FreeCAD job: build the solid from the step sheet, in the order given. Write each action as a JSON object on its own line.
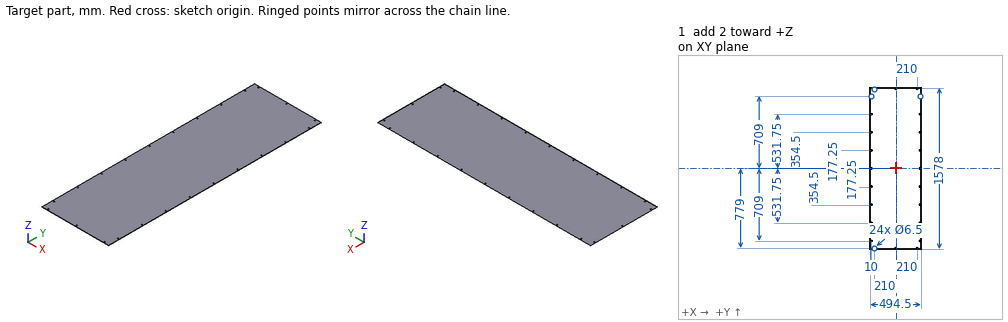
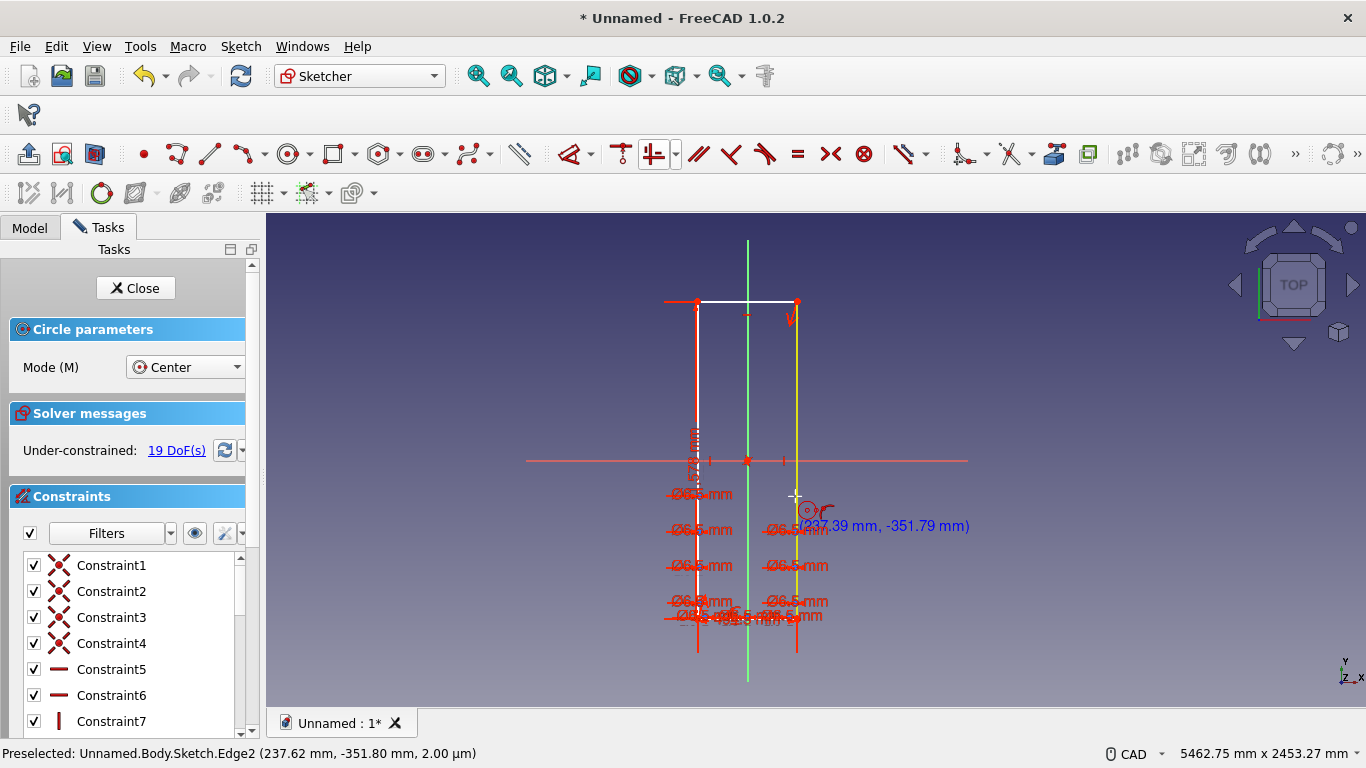
{"action": "scroll", "coordinate": [795, 496], "scroll_direction": "up", "scroll_amount": 11}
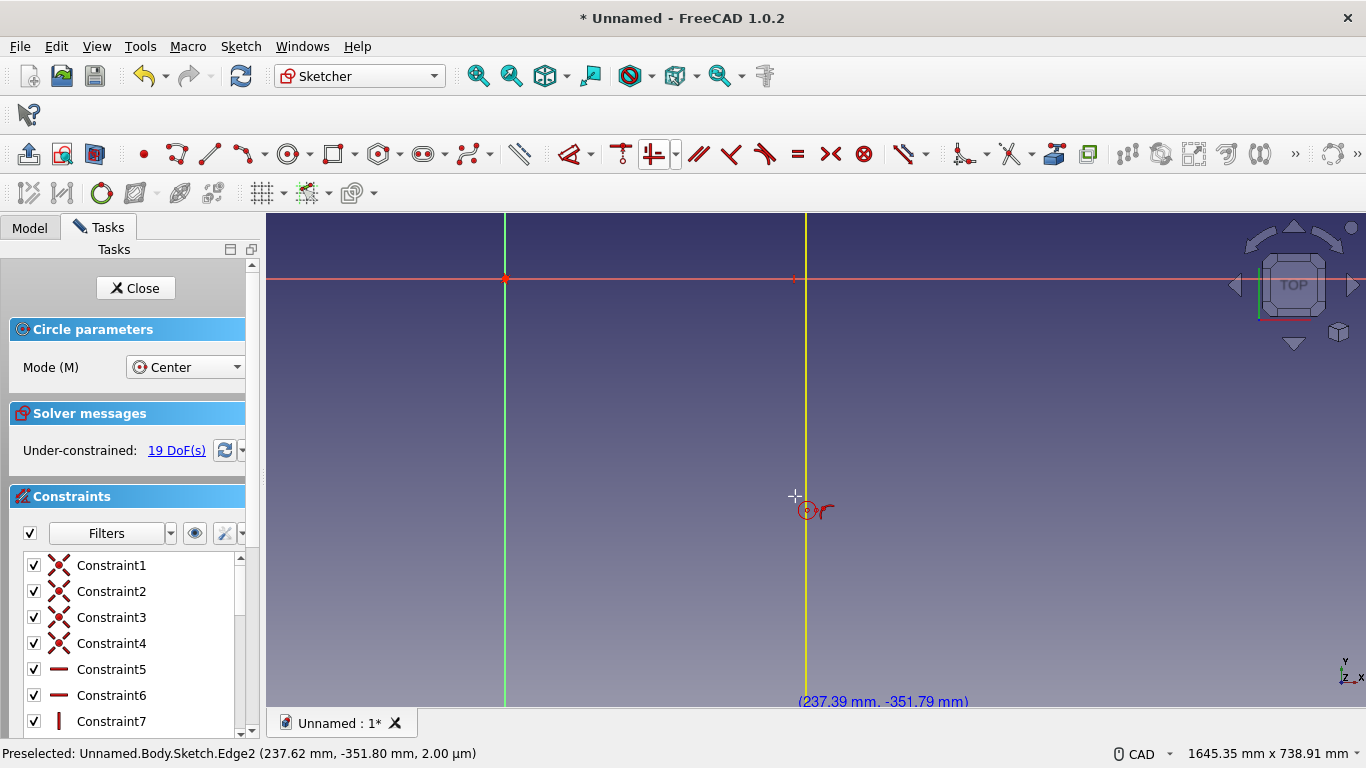
{"action": "left_click", "coordinate": [794, 493]}
{"action": "mouse_move", "coordinate": [790, 489]}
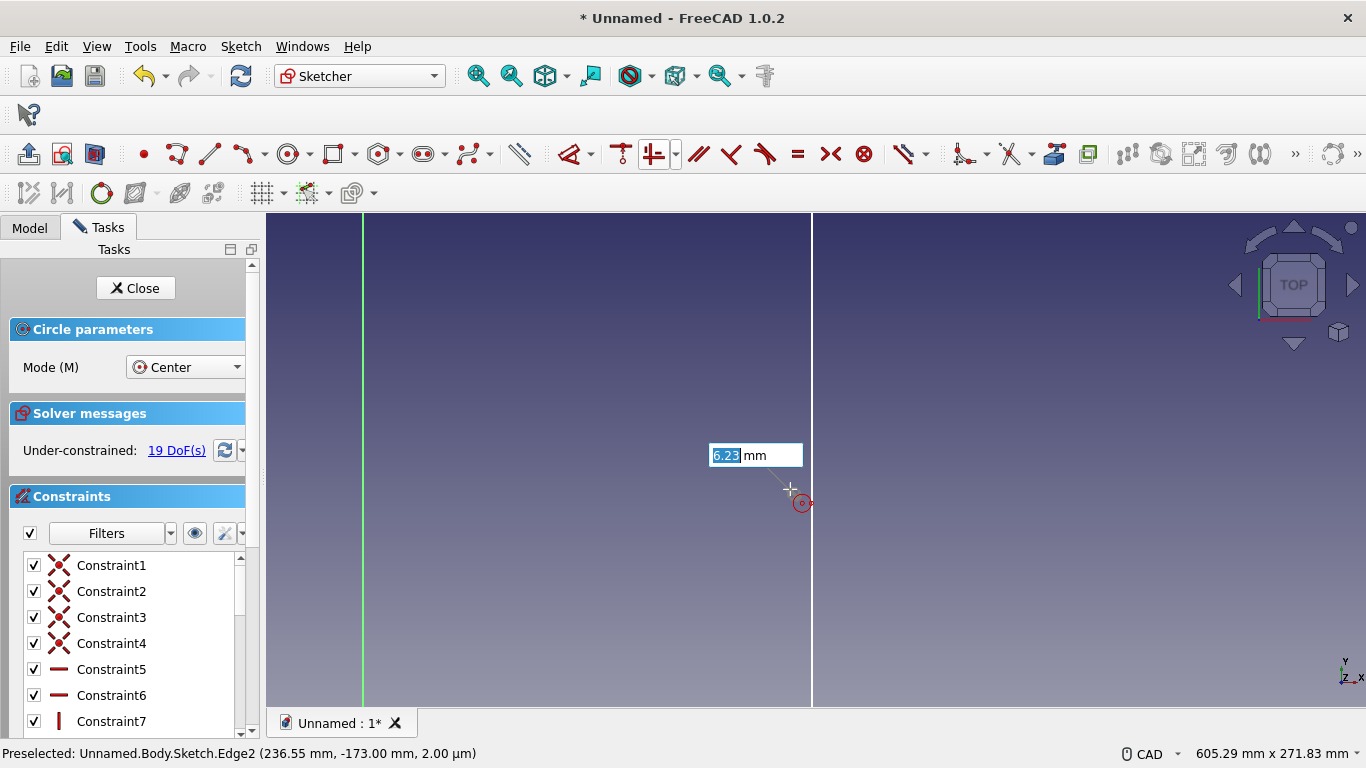
{"action": "type", "text": "6.5"}
{"action": "key", "text": "Return"}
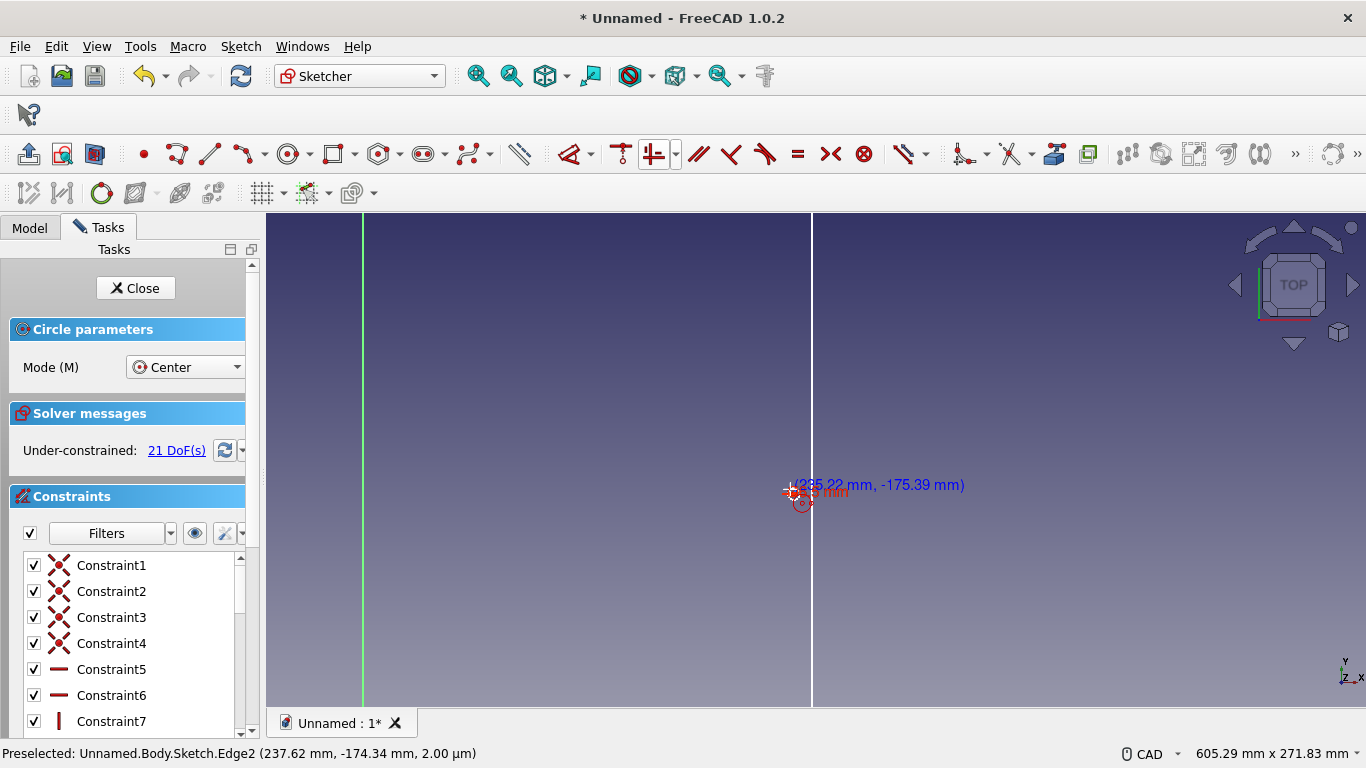
{"action": "scroll", "coordinate": [795, 496], "scroll_direction": "down", "scroll_amount": 11}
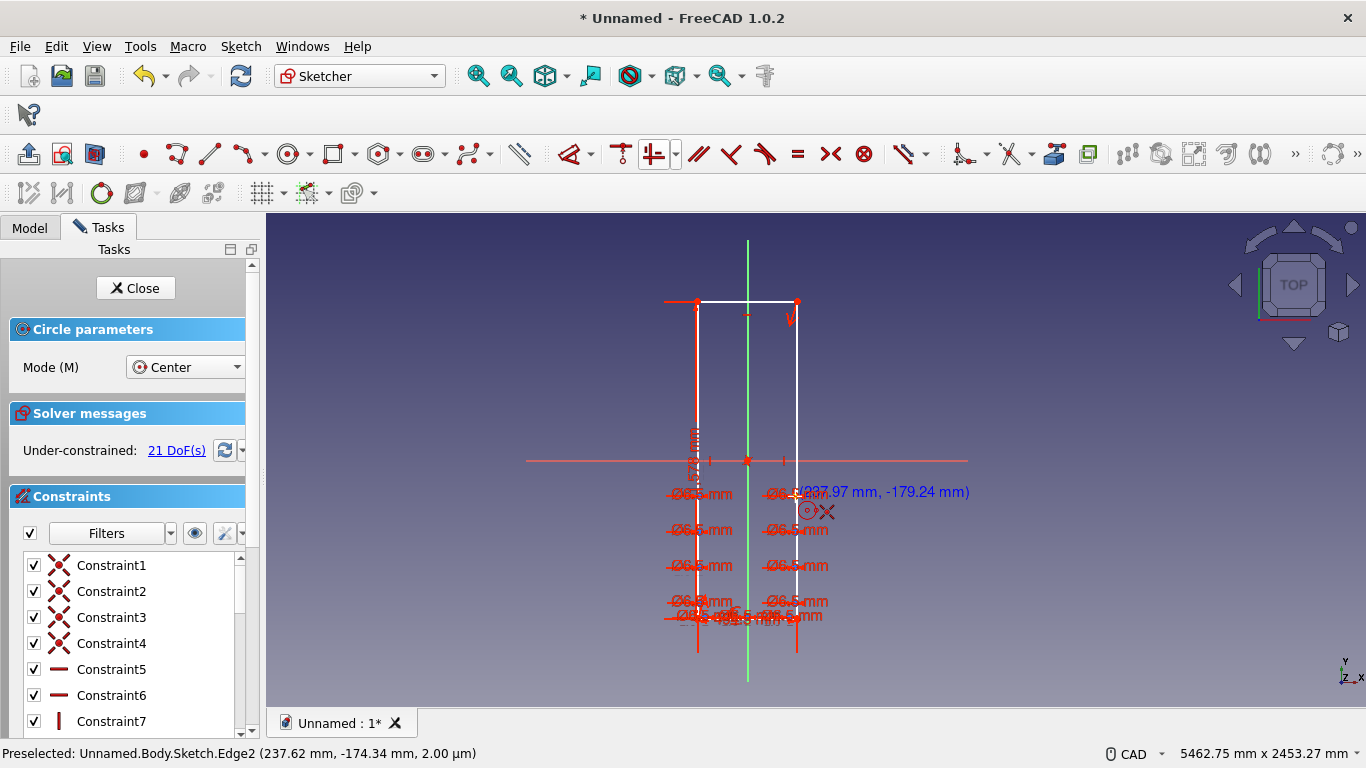
{"action": "scroll", "coordinate": [700, 461], "scroll_direction": "up", "scroll_amount": 18}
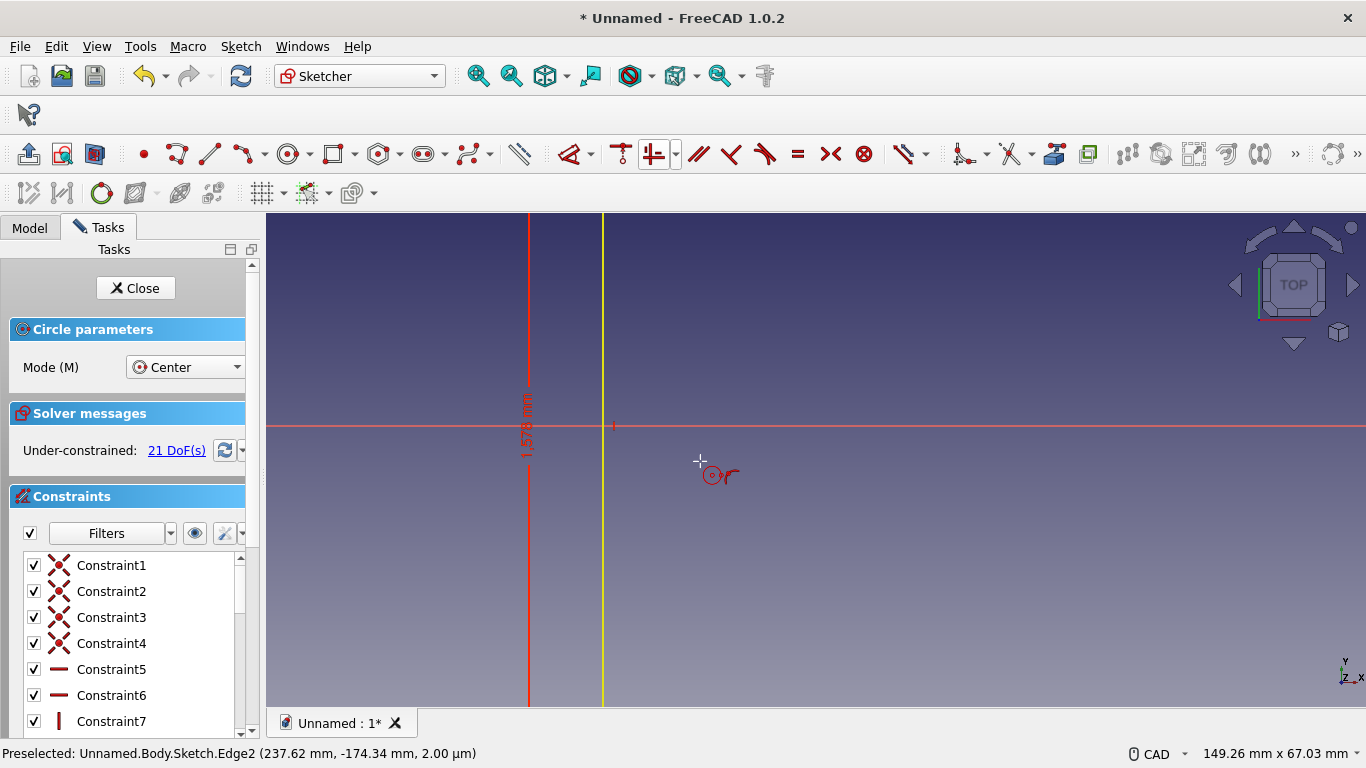
{"action": "scroll", "coordinate": [700, 461], "scroll_direction": "down", "scroll_amount": 18}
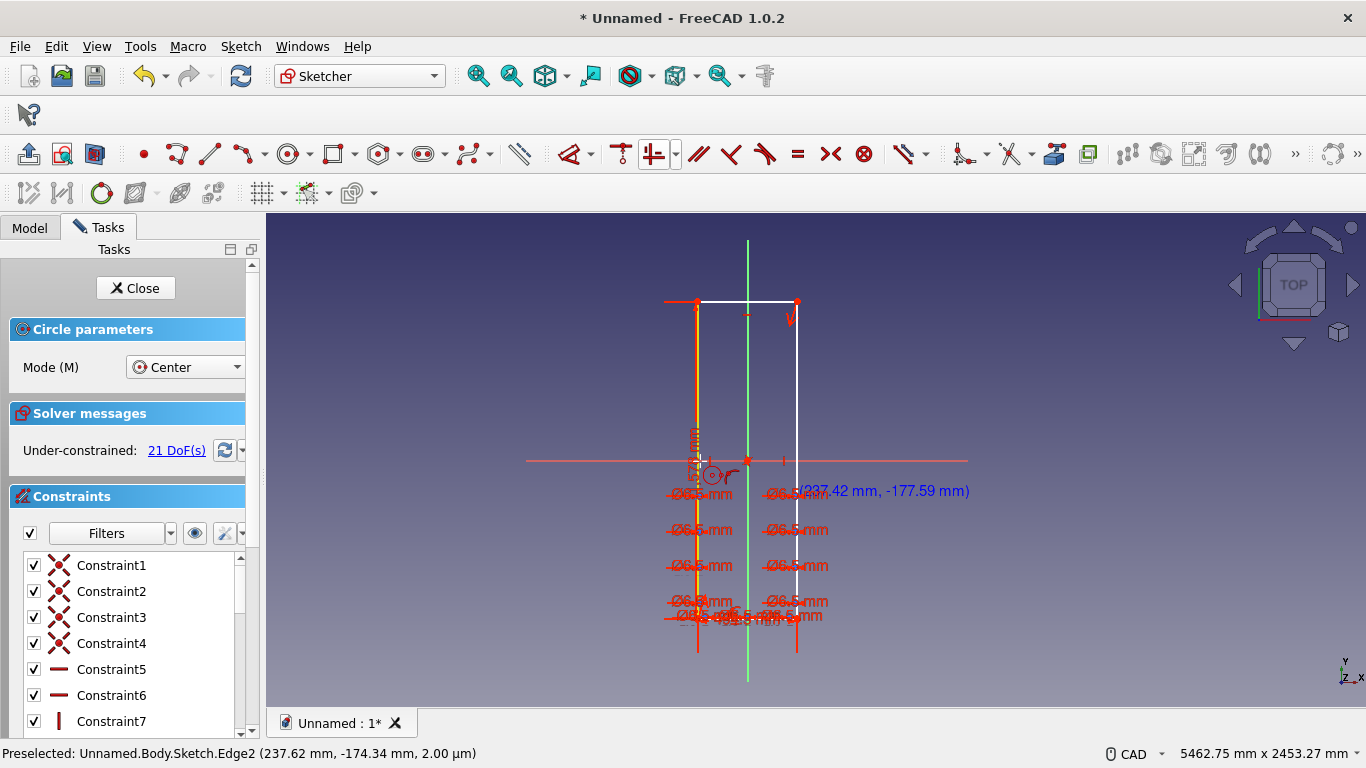
{"action": "scroll", "coordinate": [700, 461], "scroll_direction": "up", "scroll_amount": 11}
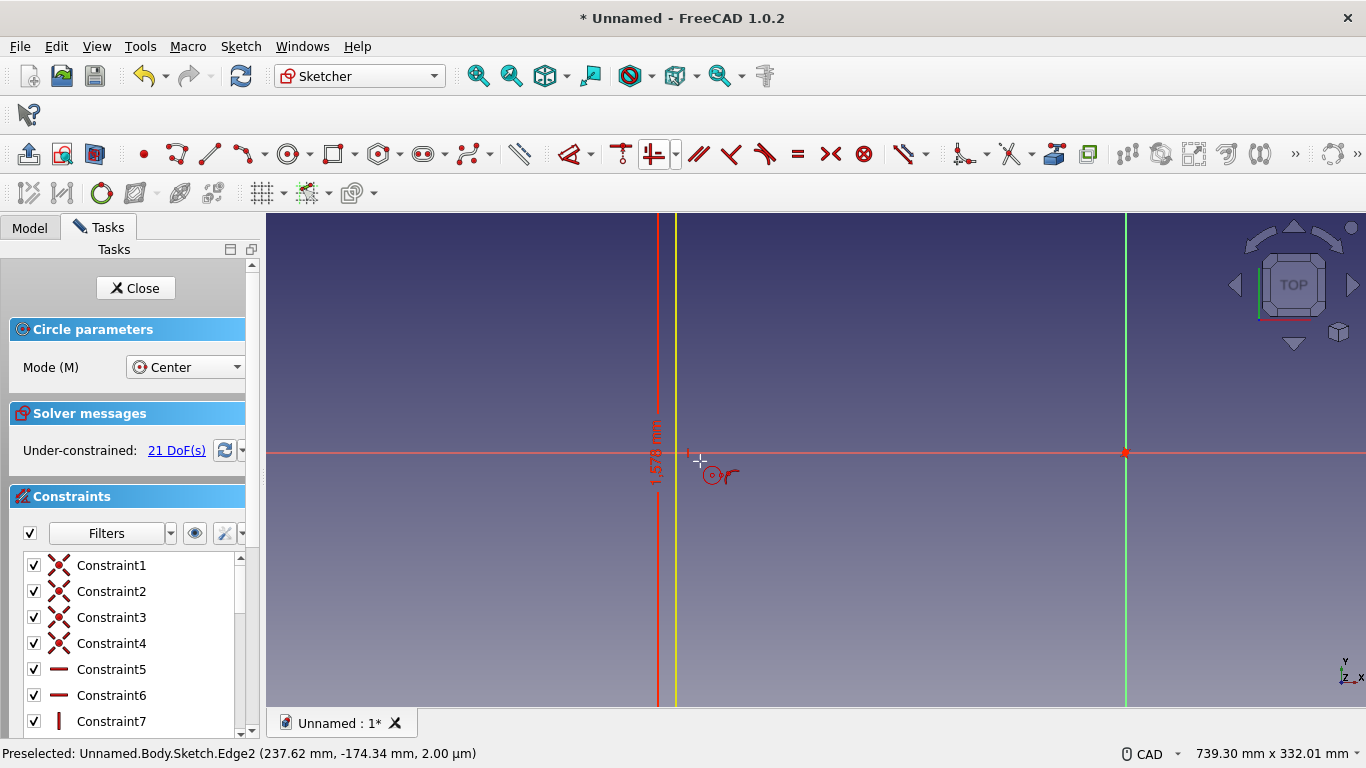
{"action": "left_click", "coordinate": [694, 453]}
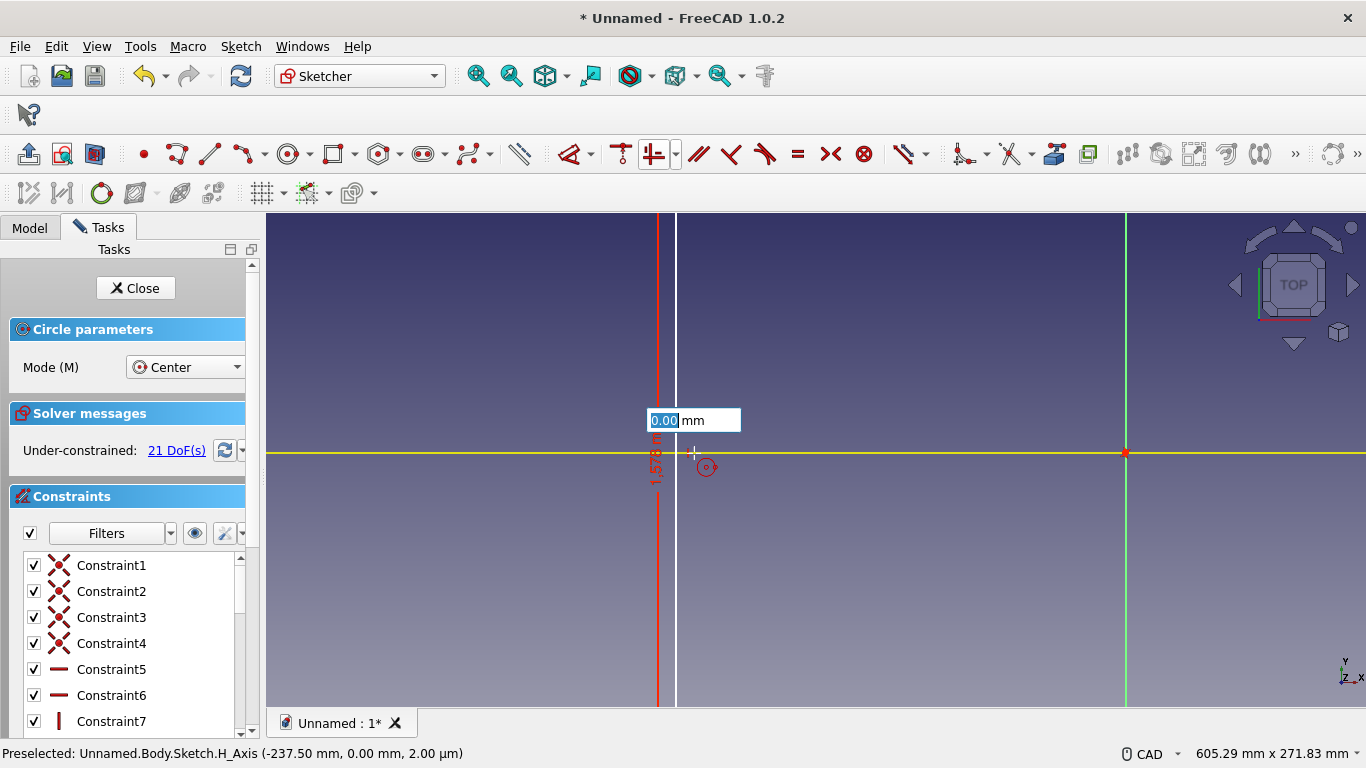
{"action": "scroll", "coordinate": [692, 458], "scroll_direction": "up", "scroll_amount": 6}
{"action": "mouse_move", "coordinate": [693, 458]}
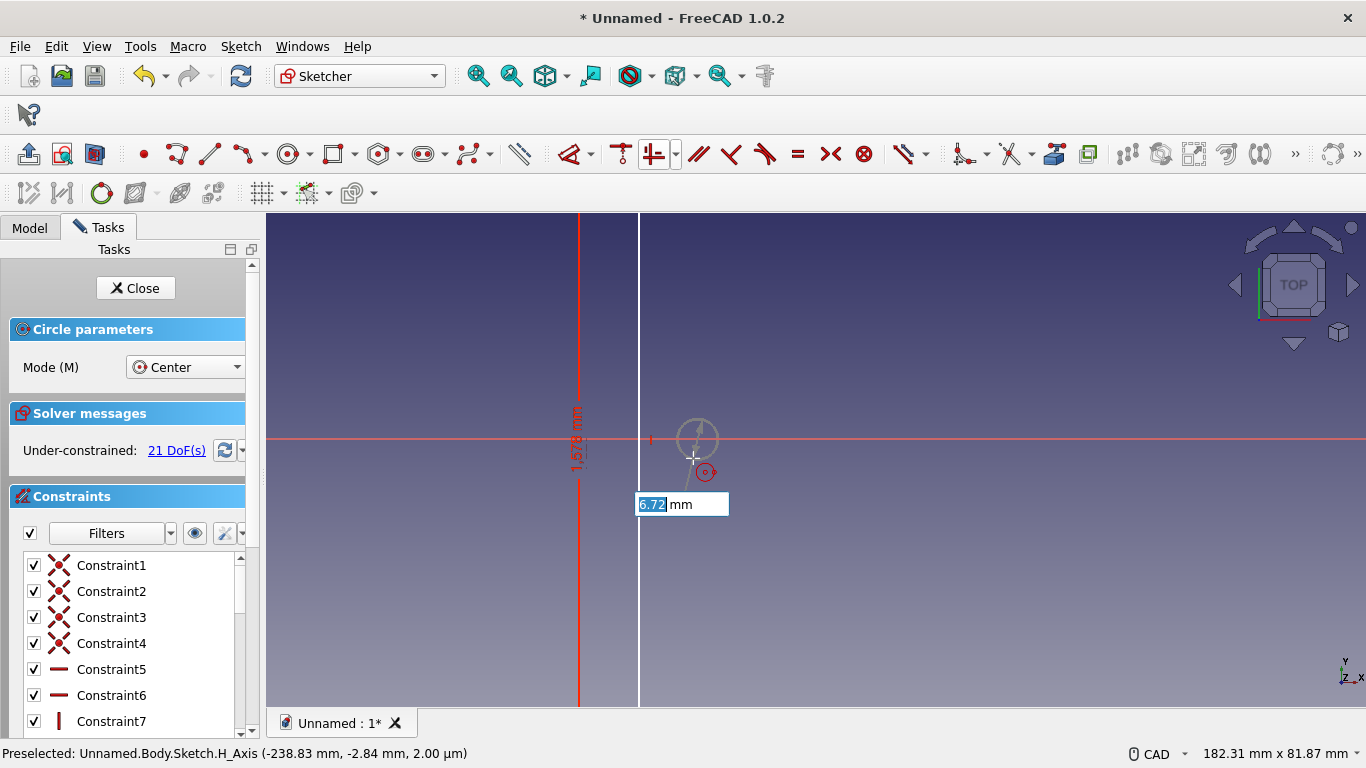
{"action": "type", "text": "6.5"}
{"action": "key", "text": "Return"}